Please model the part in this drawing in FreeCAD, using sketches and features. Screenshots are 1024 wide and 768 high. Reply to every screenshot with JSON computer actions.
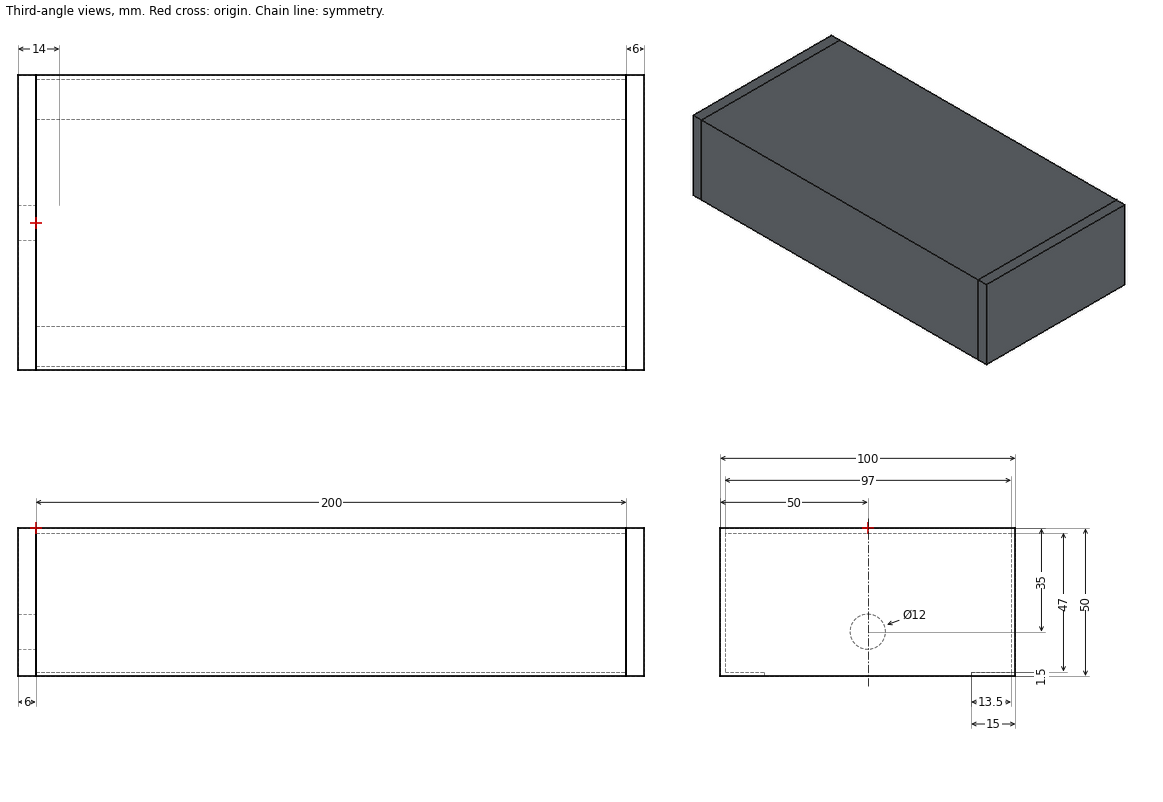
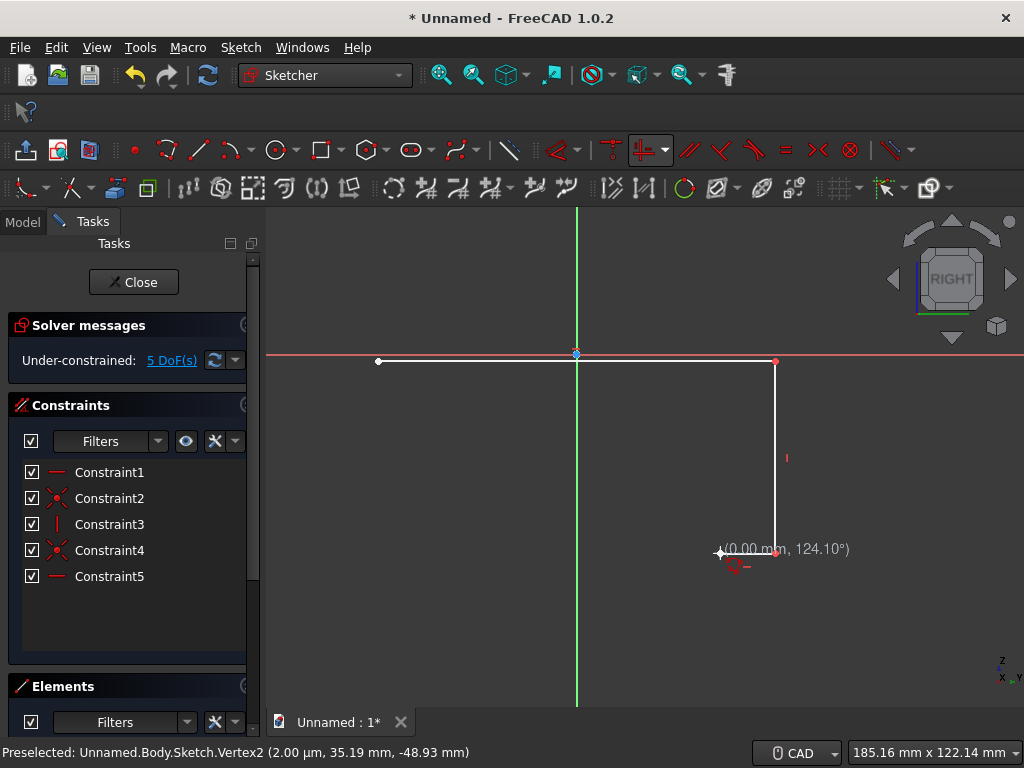
{"action": "scroll", "coordinate": [720, 559], "scroll_direction": "up", "scroll_amount": 5}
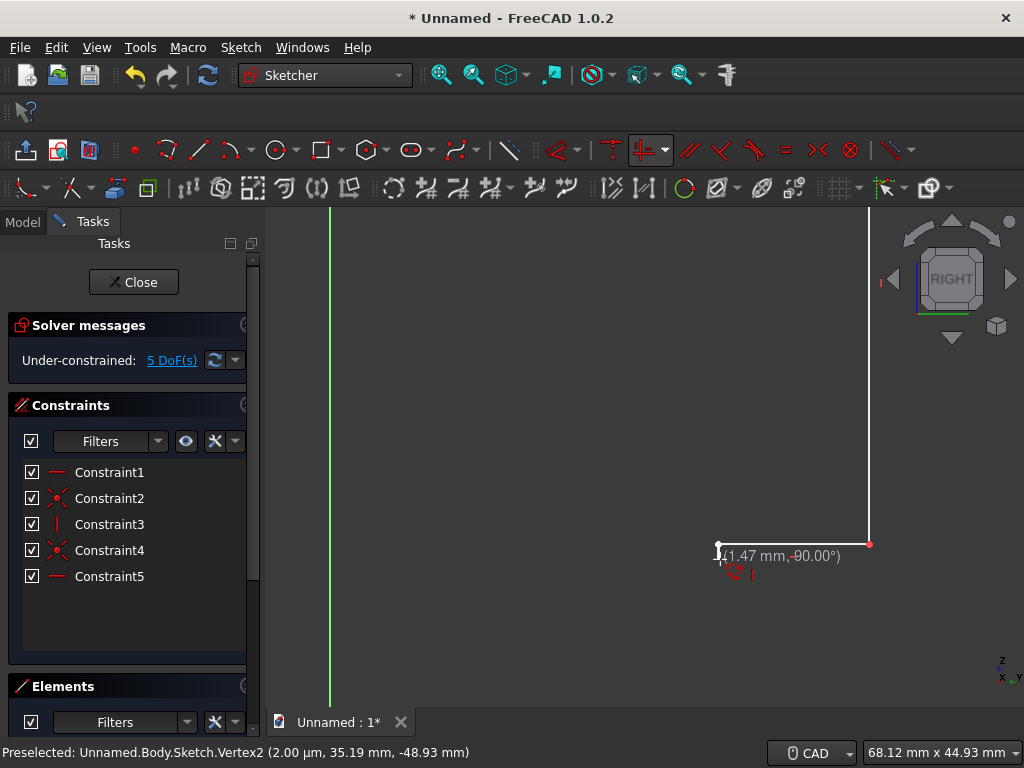
{"action": "left_click", "coordinate": [719, 559]}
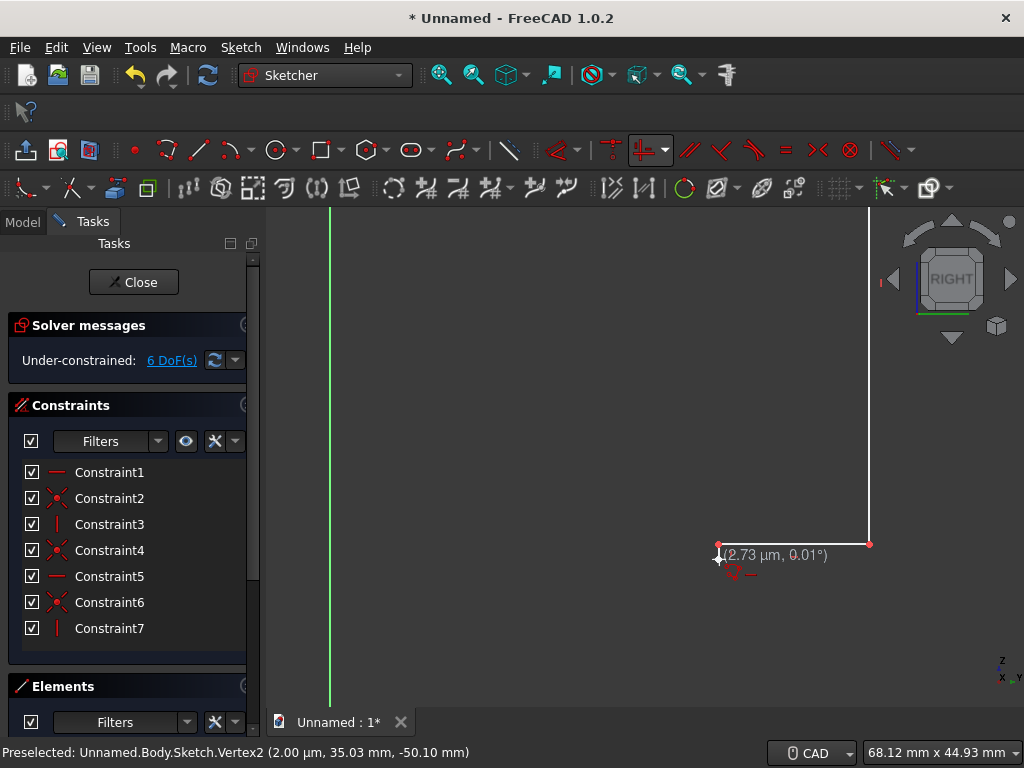
{"action": "scroll", "coordinate": [720, 560], "scroll_direction": "down", "scroll_amount": 5}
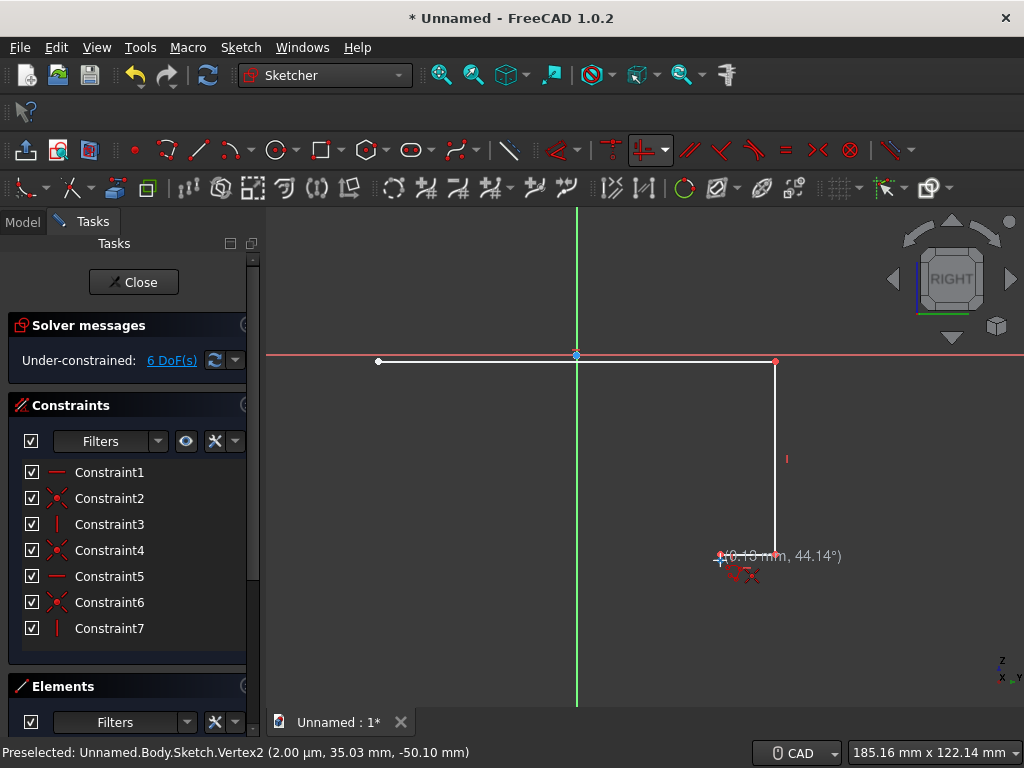
{"action": "scroll", "coordinate": [782, 560], "scroll_direction": "up", "scroll_amount": 4}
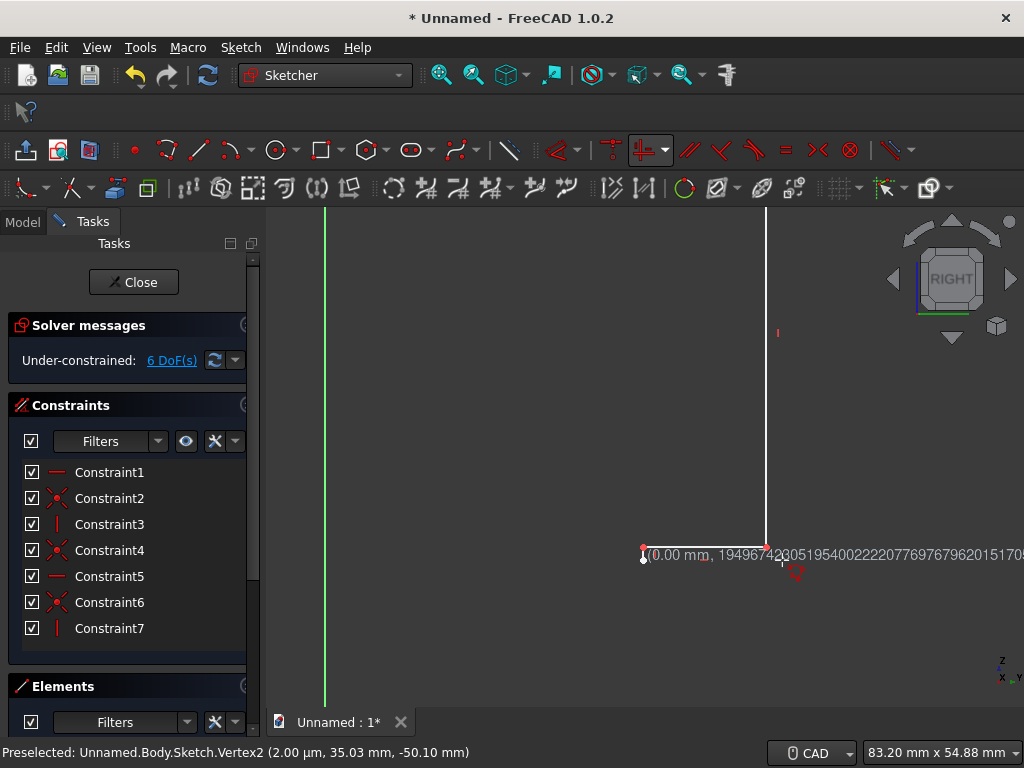
{"action": "left_click", "coordinate": [780, 559]}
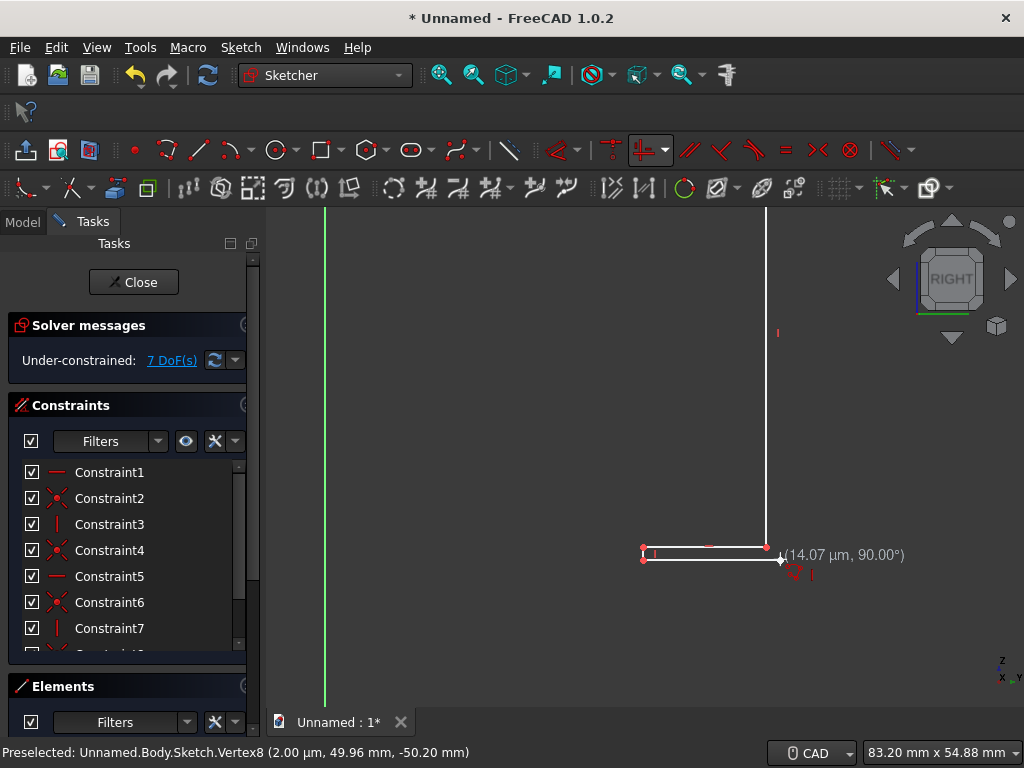
{"action": "scroll", "coordinate": [782, 559], "scroll_direction": "down", "scroll_amount": 4}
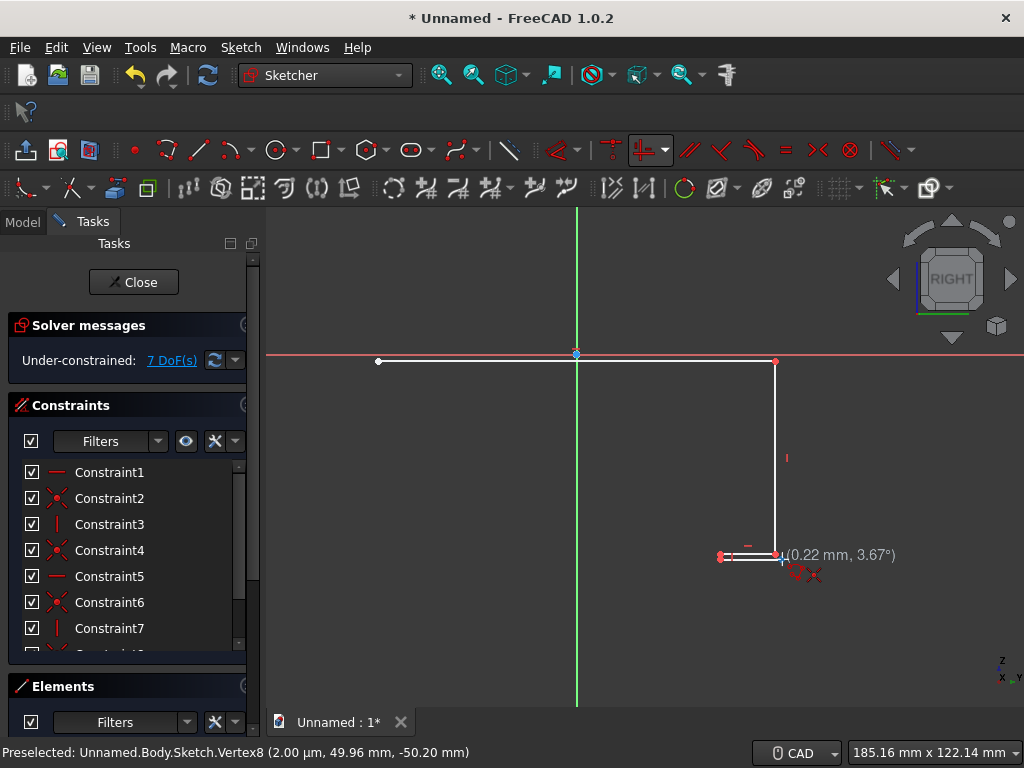
{"action": "scroll", "coordinate": [782, 355], "scroll_direction": "up", "scroll_amount": 4}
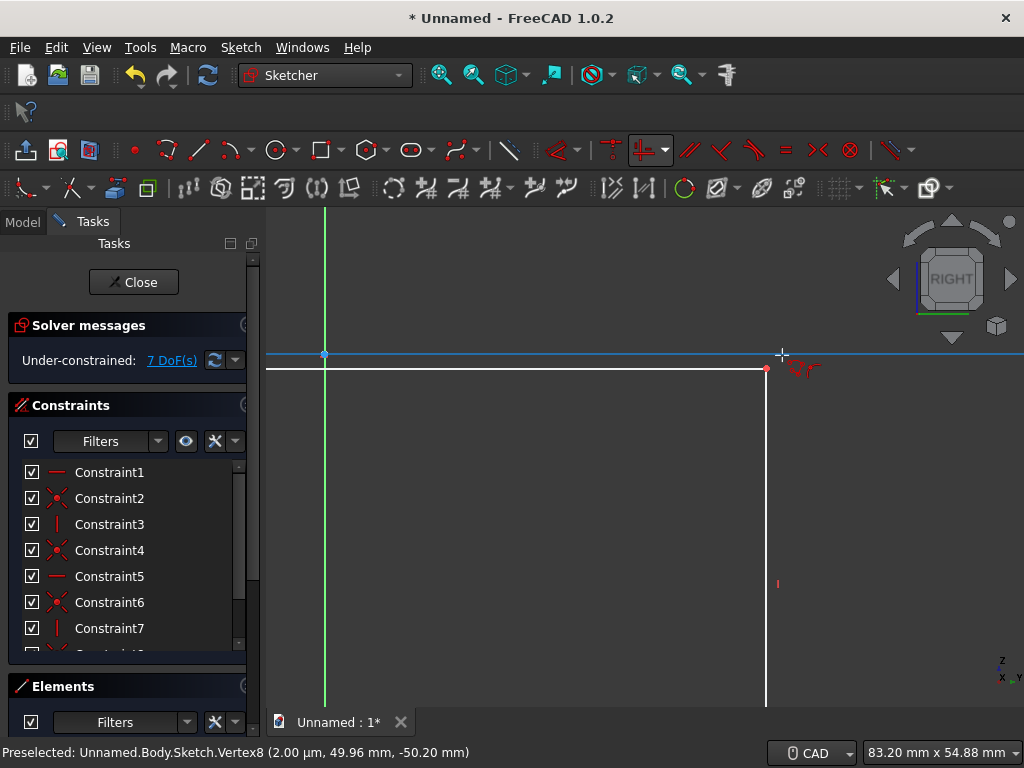
{"action": "left_click", "coordinate": [780, 354]}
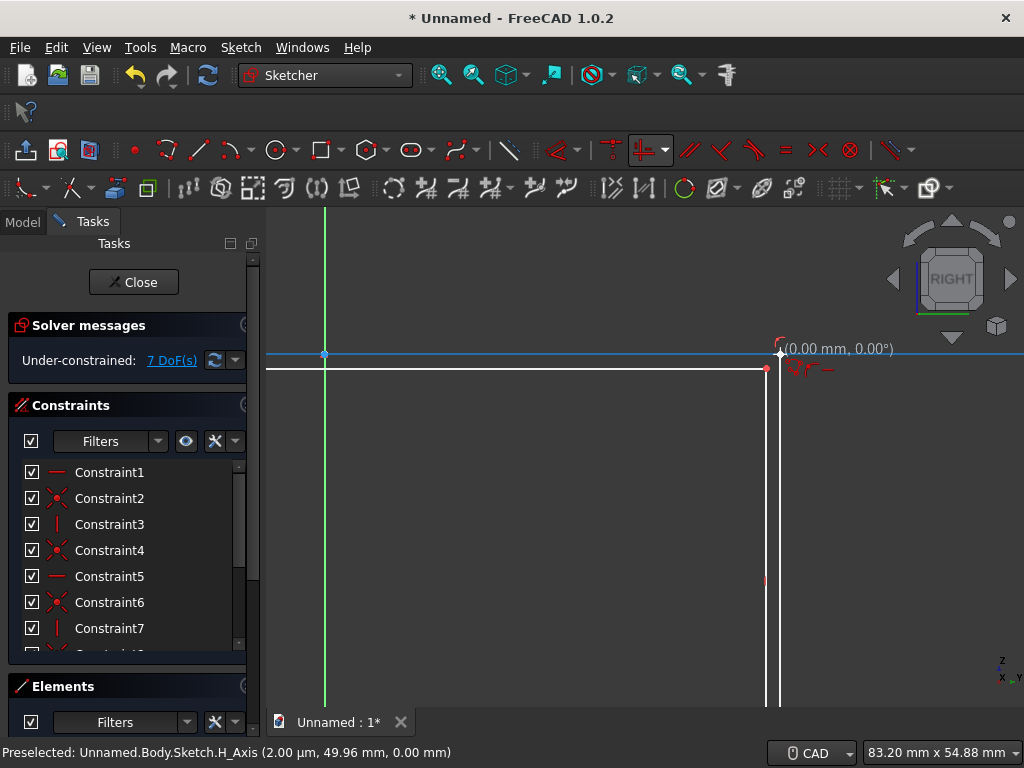
{"action": "scroll", "coordinate": [782, 355], "scroll_direction": "down", "scroll_amount": 4}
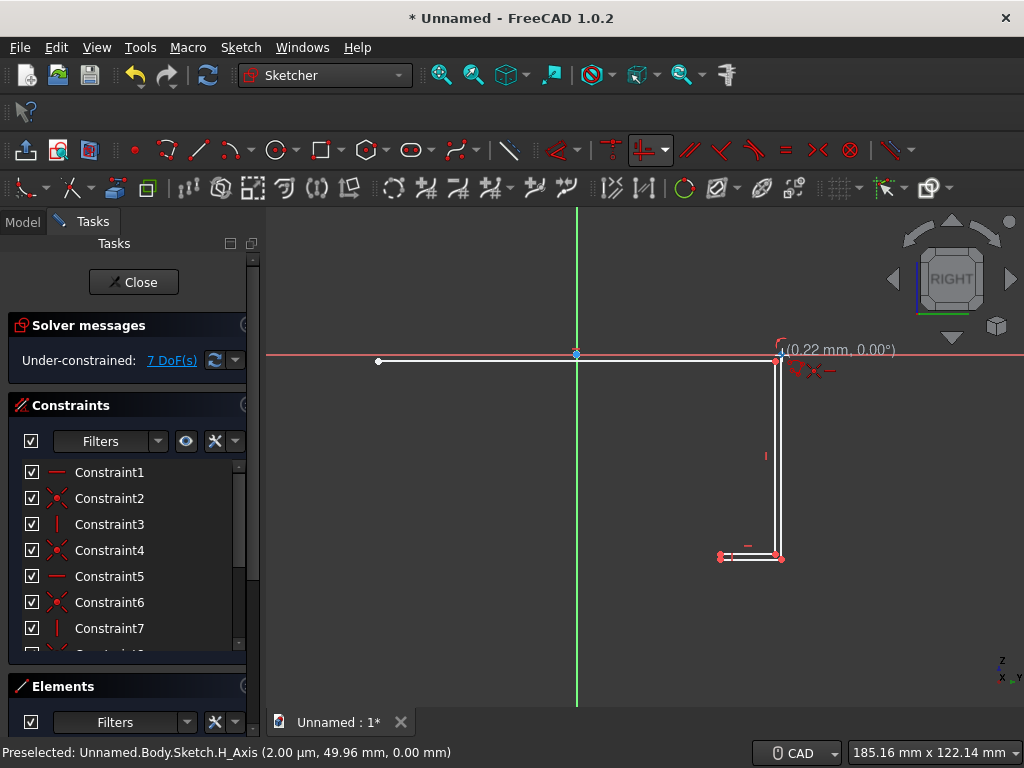
{"action": "scroll", "coordinate": [372, 355], "scroll_direction": "up", "scroll_amount": 4}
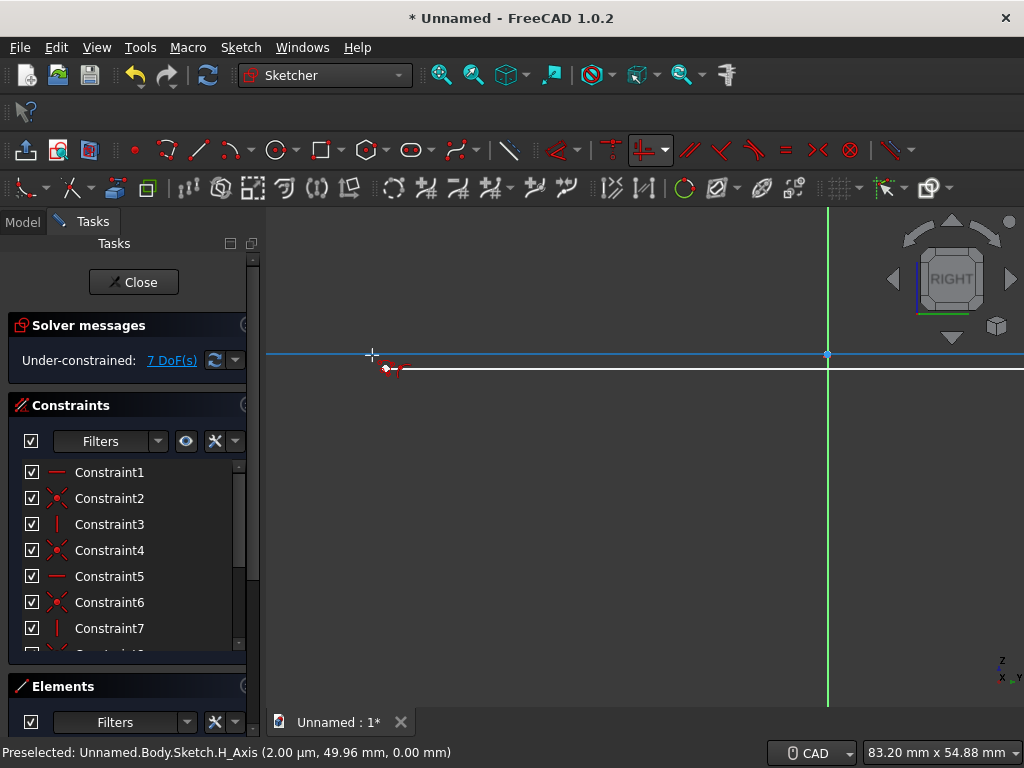
{"action": "left_click", "coordinate": [372, 363]}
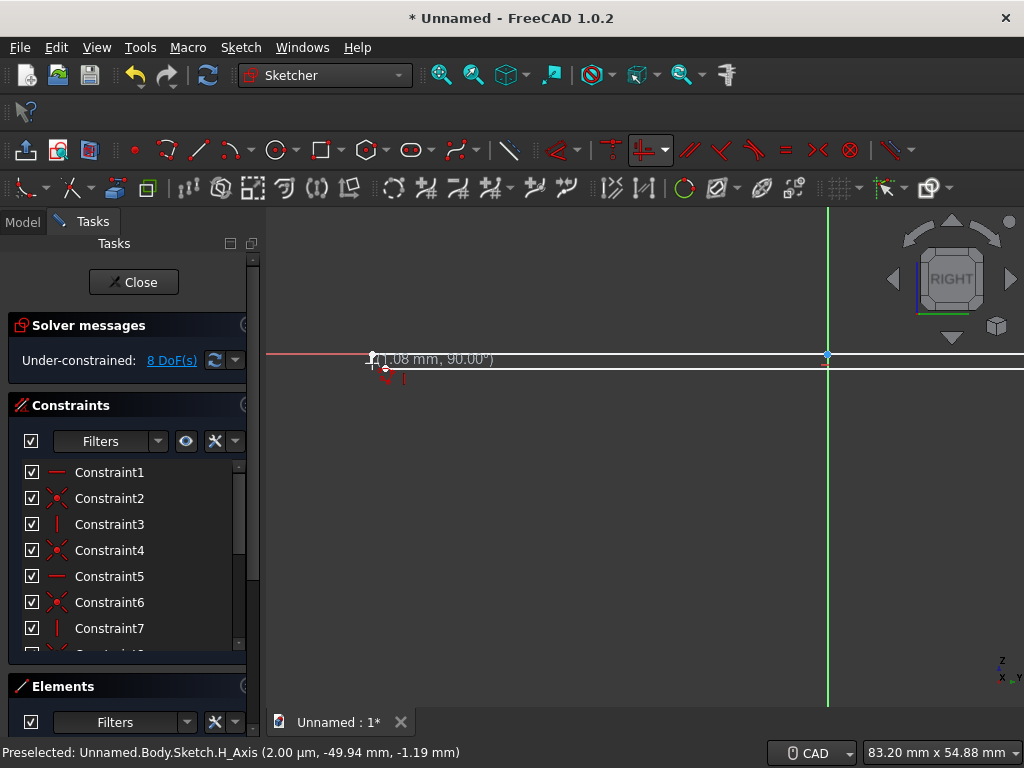
{"action": "scroll", "coordinate": [371, 355], "scroll_direction": "down", "scroll_amount": 4}